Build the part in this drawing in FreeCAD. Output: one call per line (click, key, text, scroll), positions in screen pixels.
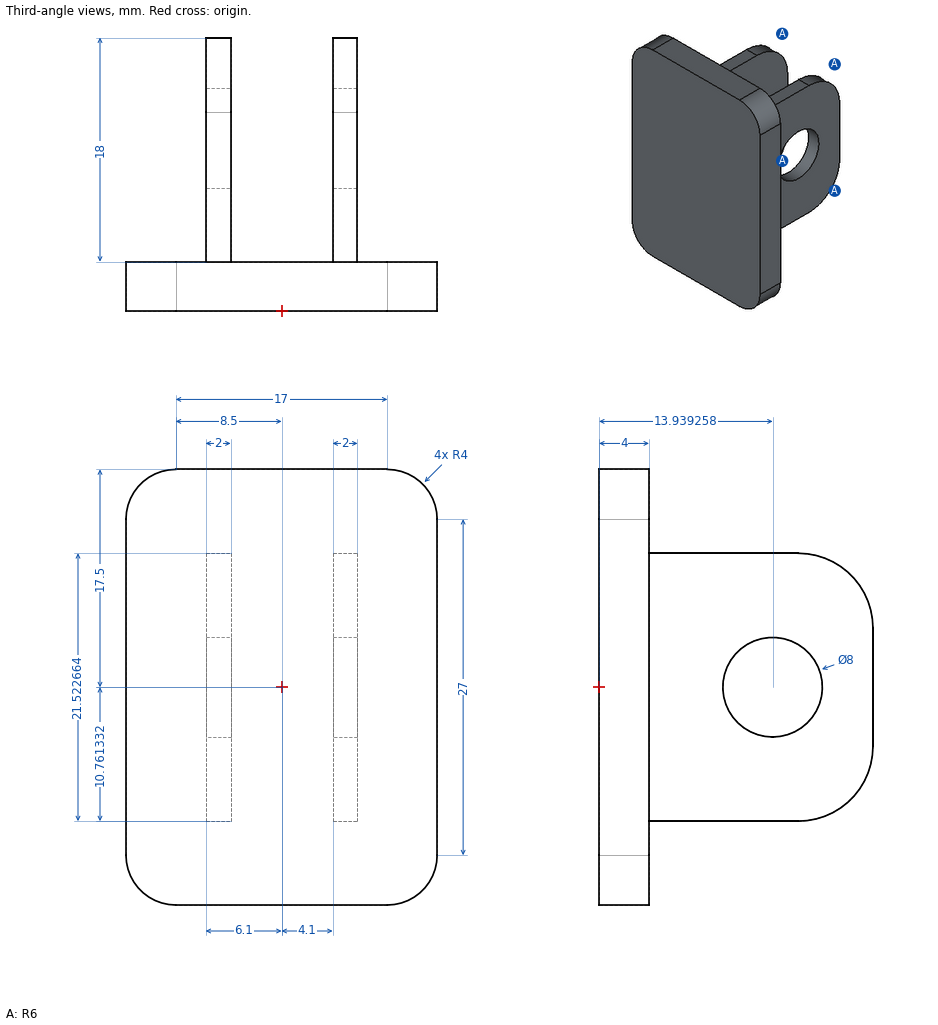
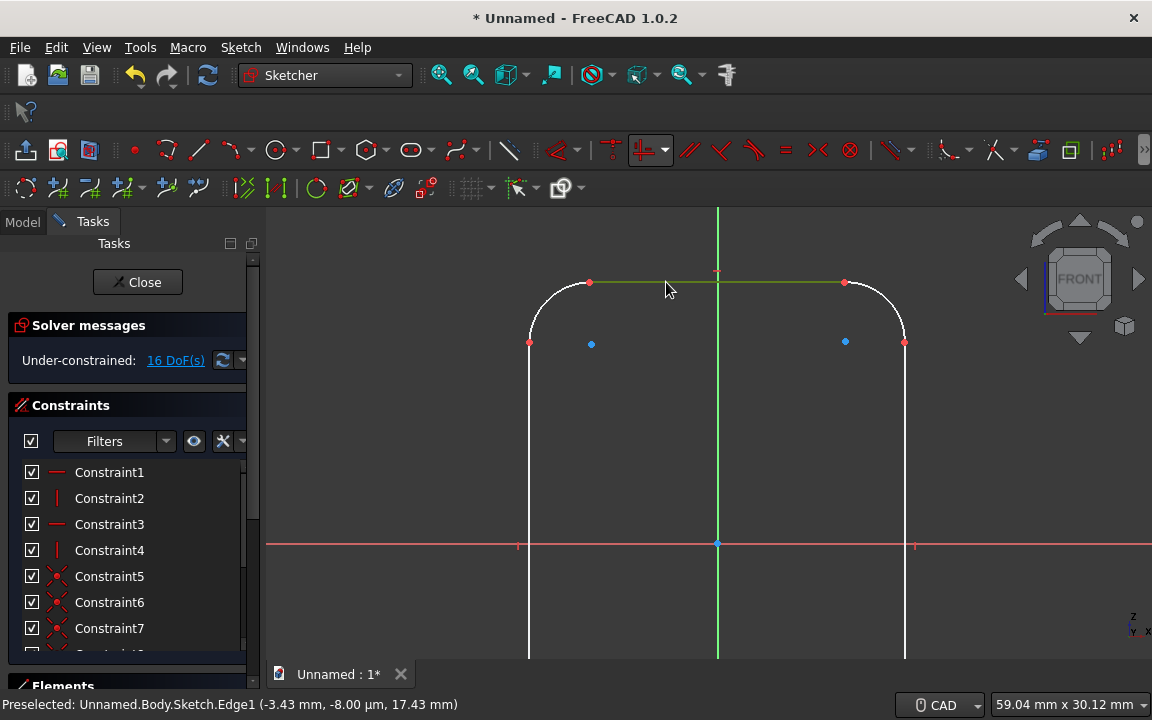
click(898, 315)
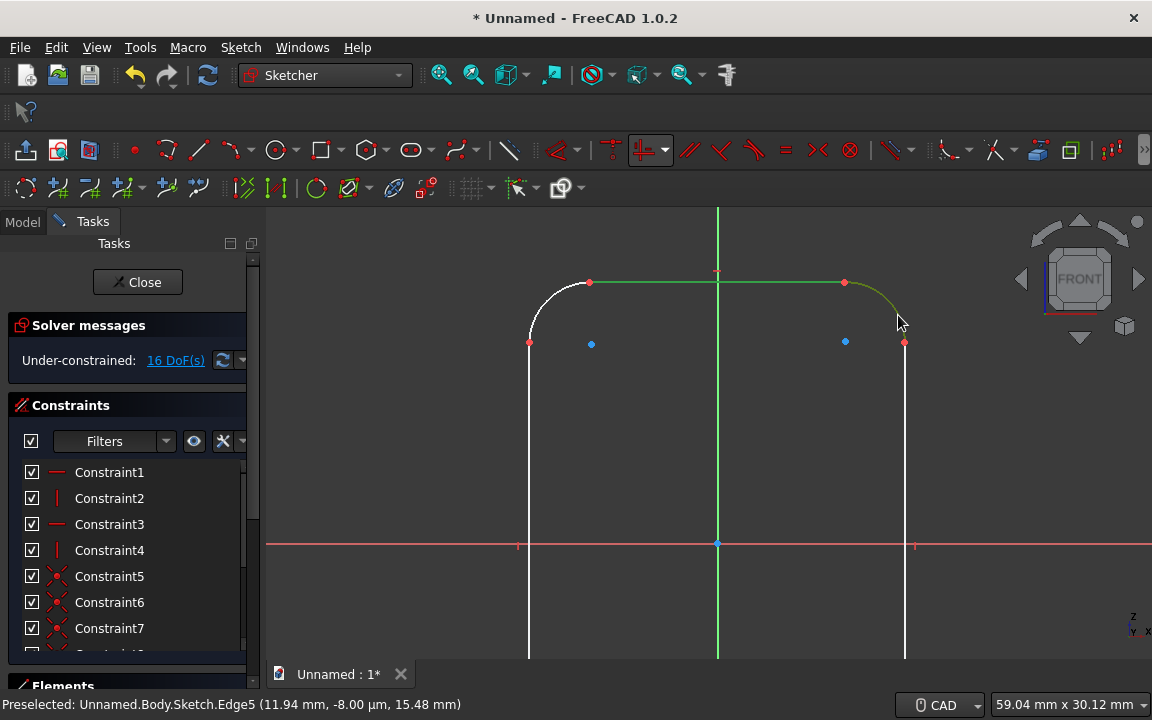
click(754, 150)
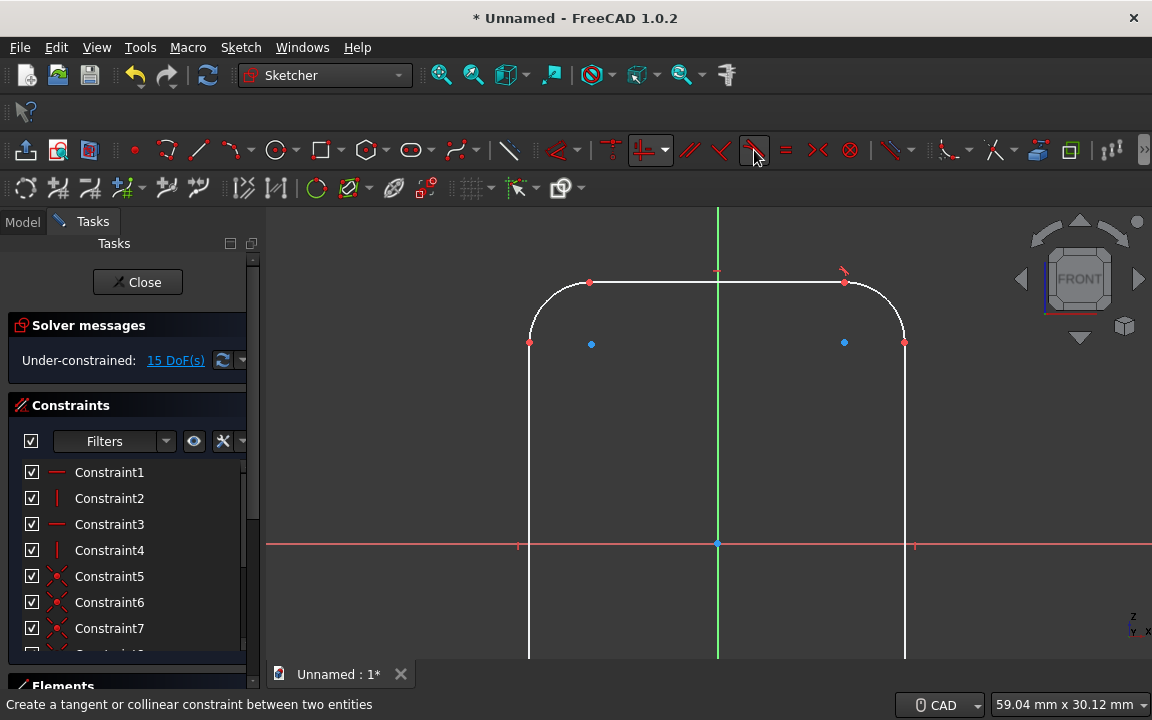
click(666, 282)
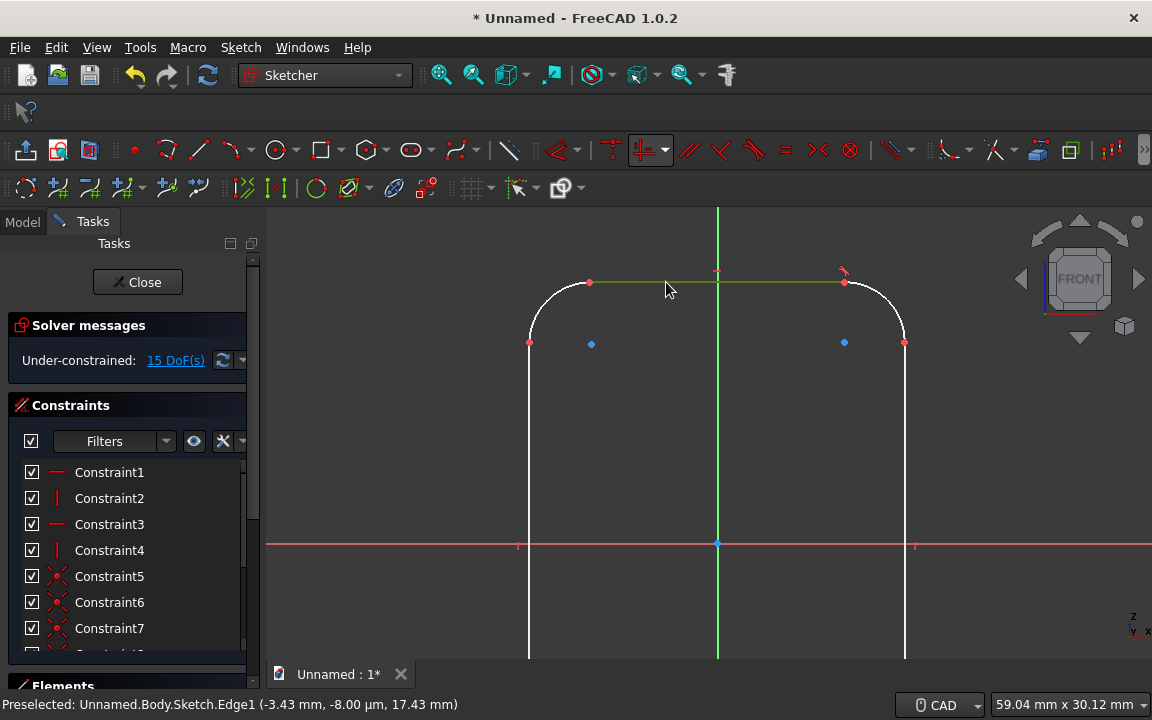
click(563, 289)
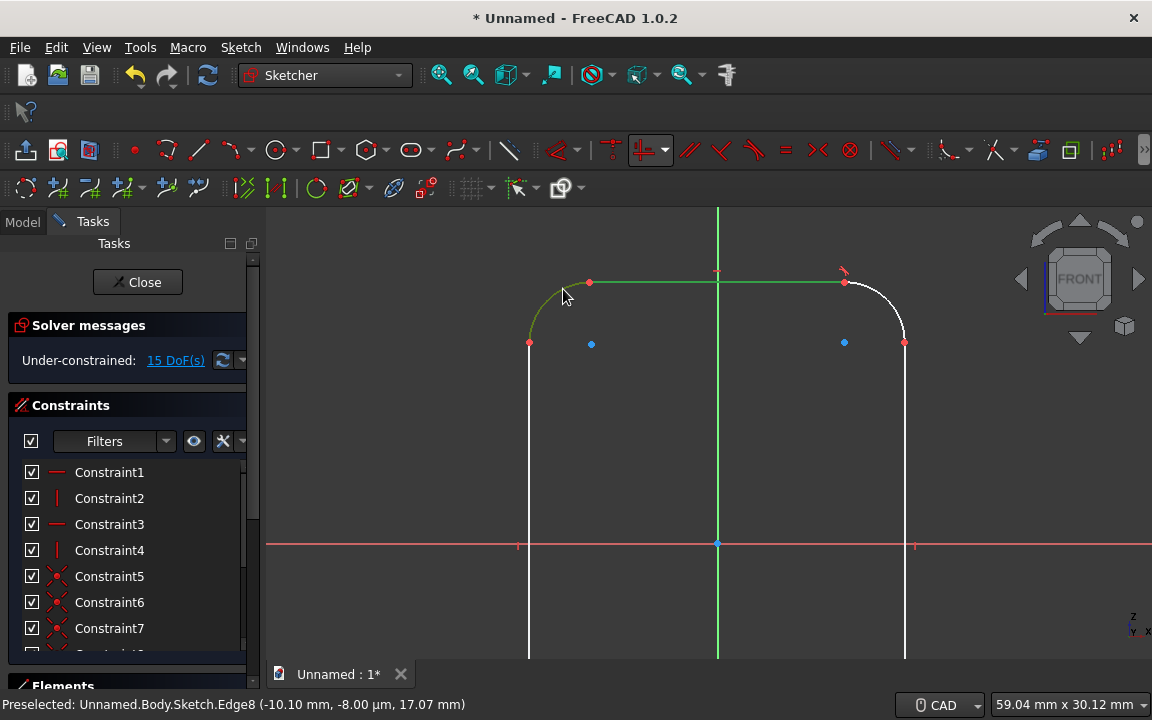
click(754, 150)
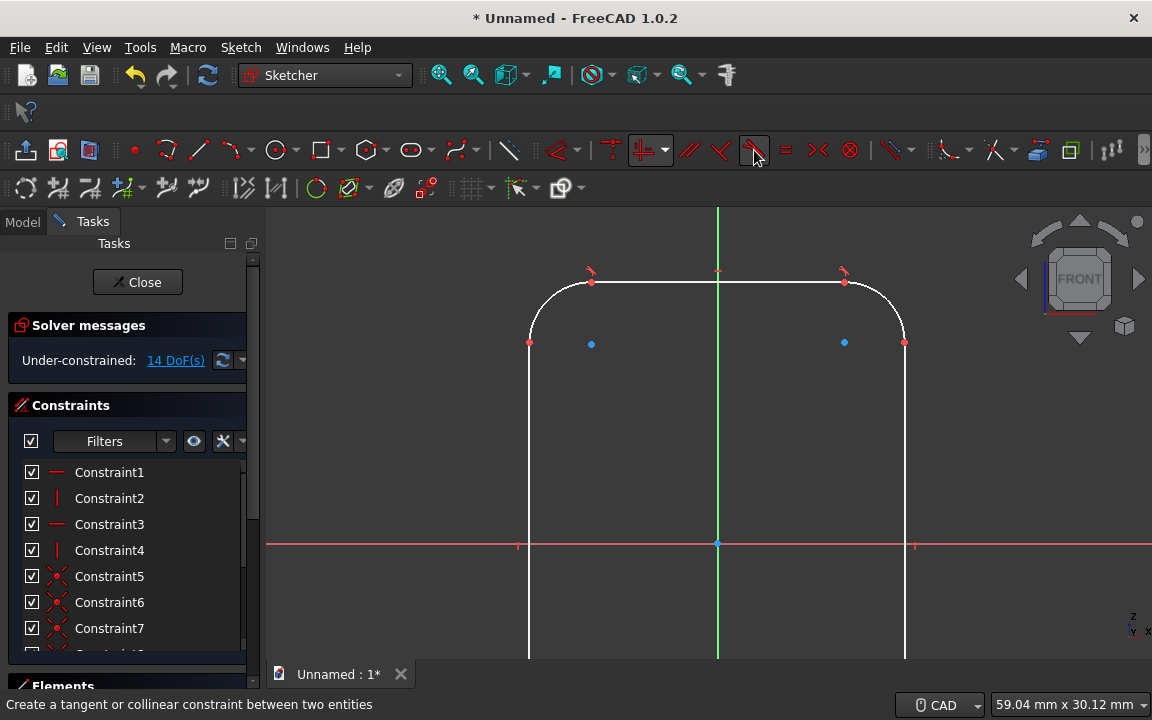
click(905, 464)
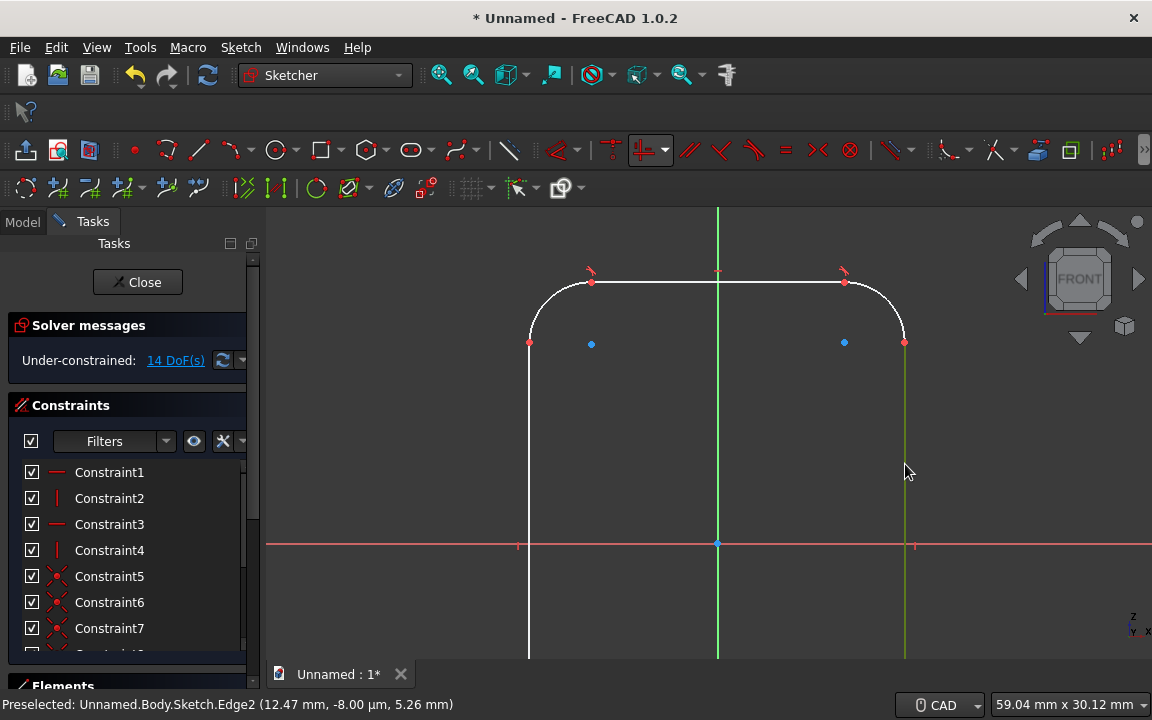
click(898, 315)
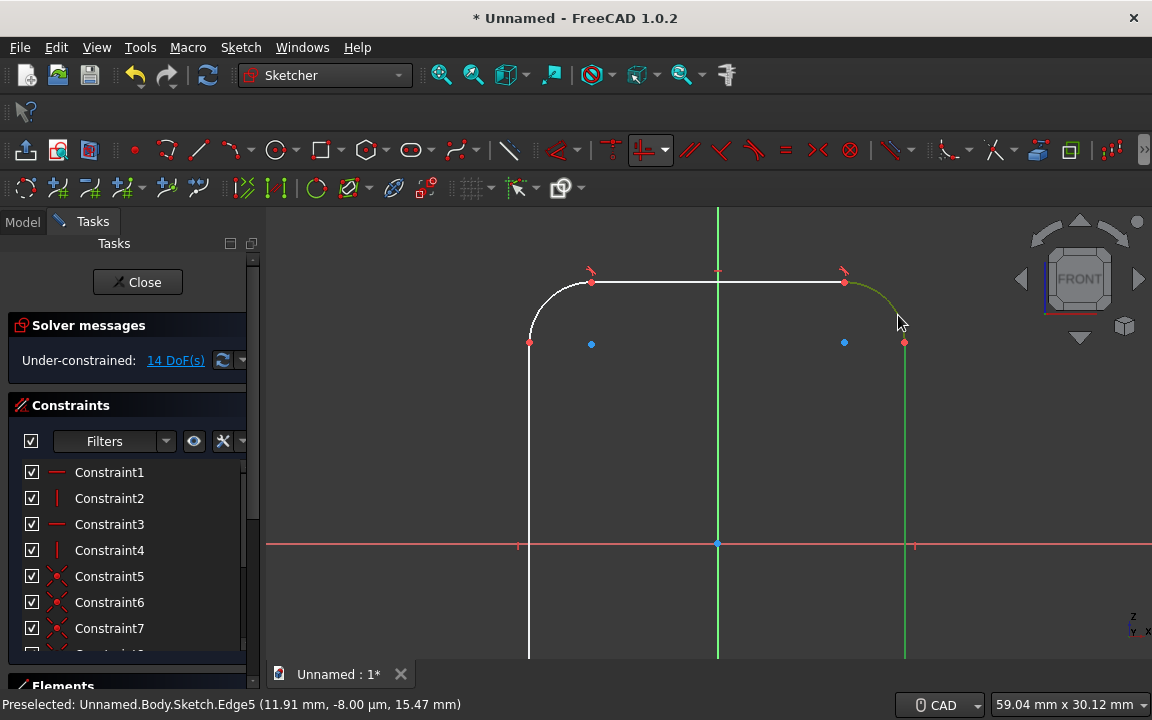
click(754, 150)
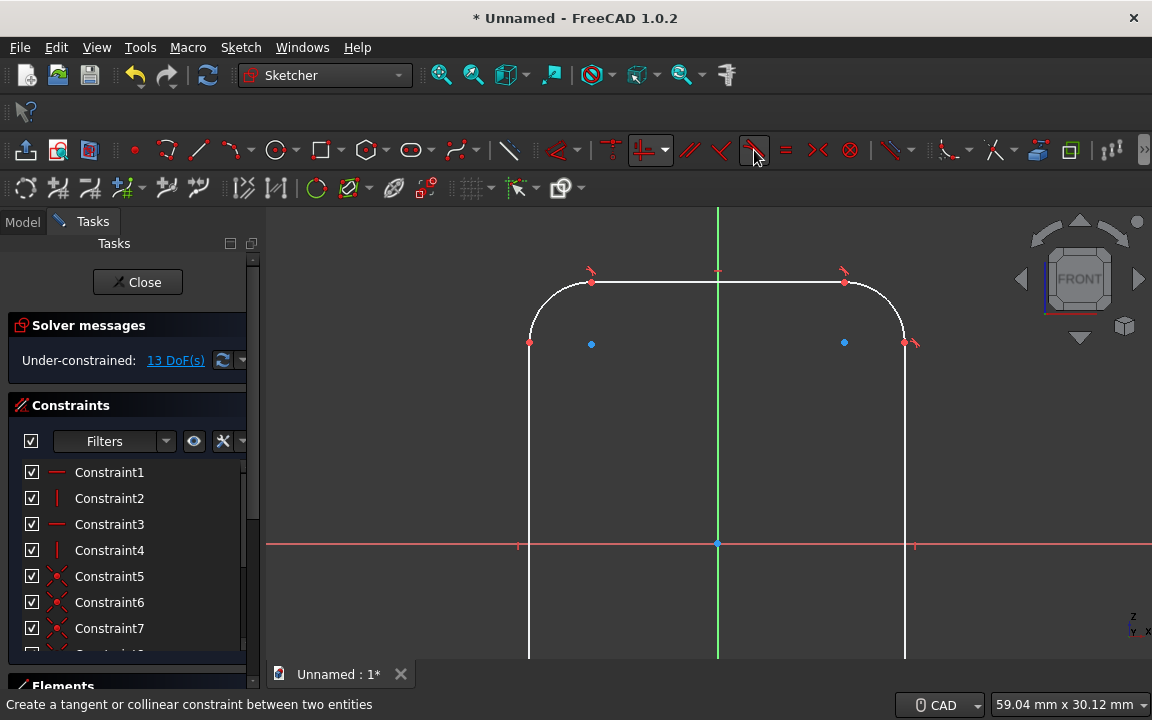
click(905, 464)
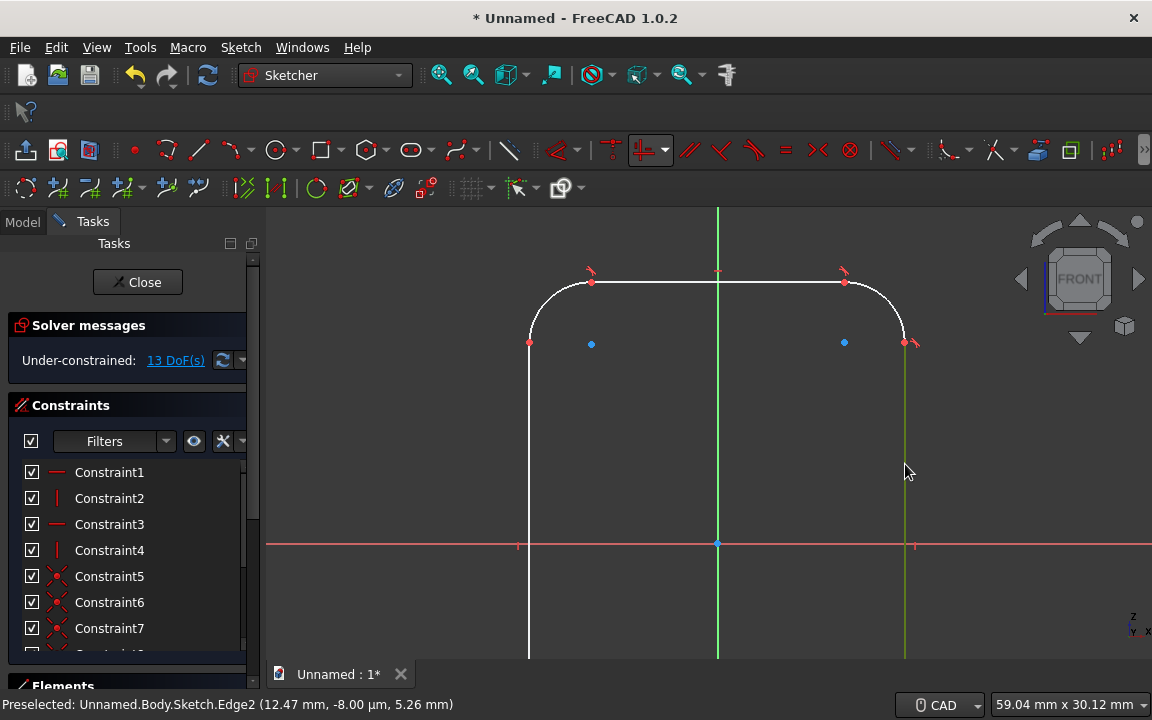
scroll(547, 298, down, 3)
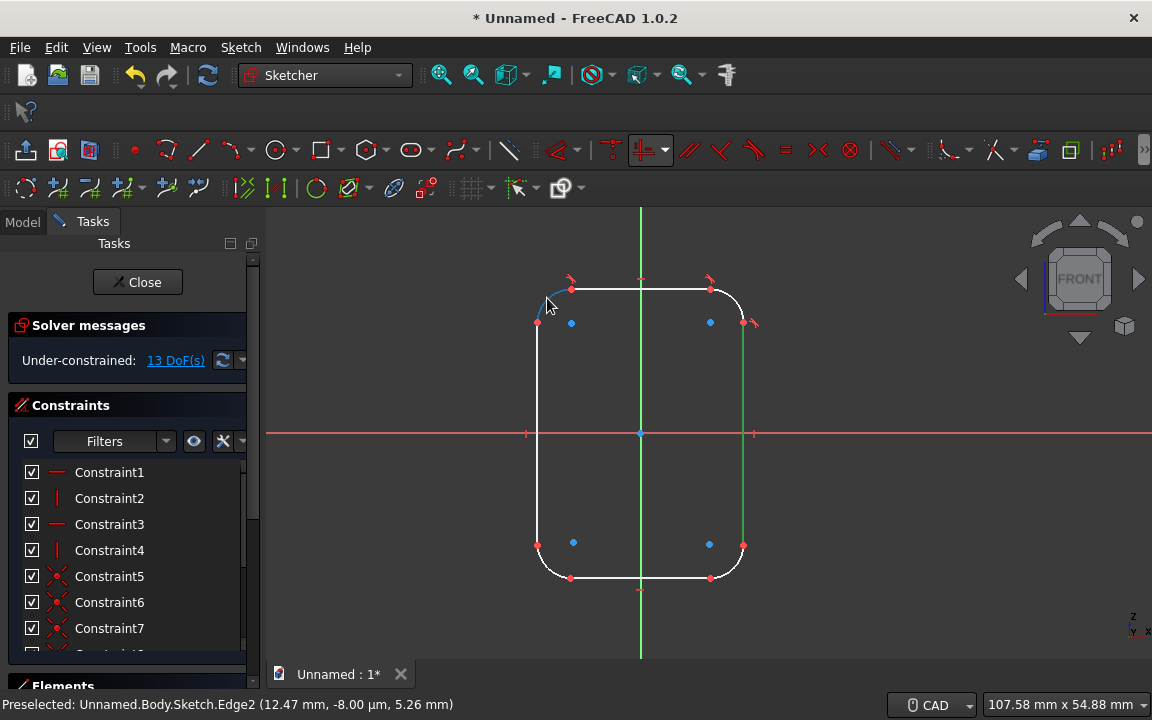
click(725, 575)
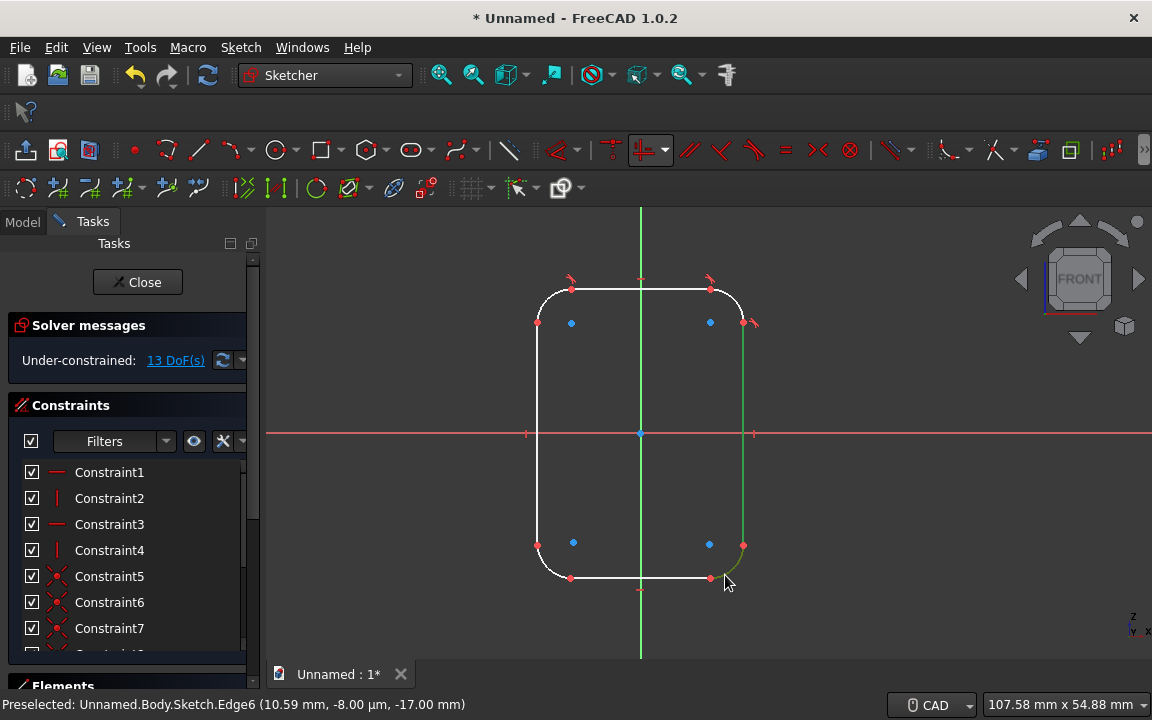
click(754, 150)